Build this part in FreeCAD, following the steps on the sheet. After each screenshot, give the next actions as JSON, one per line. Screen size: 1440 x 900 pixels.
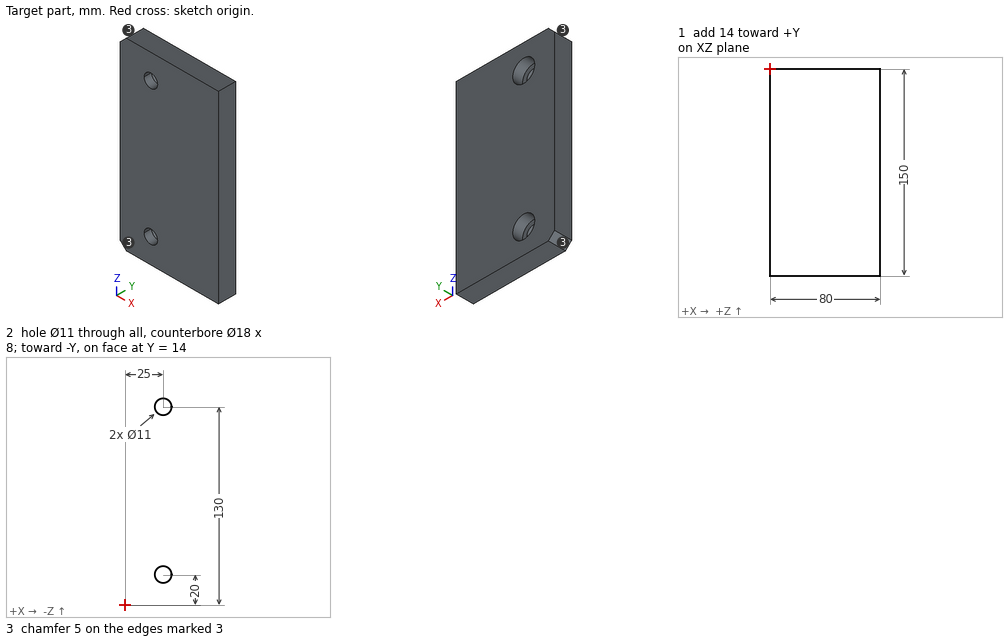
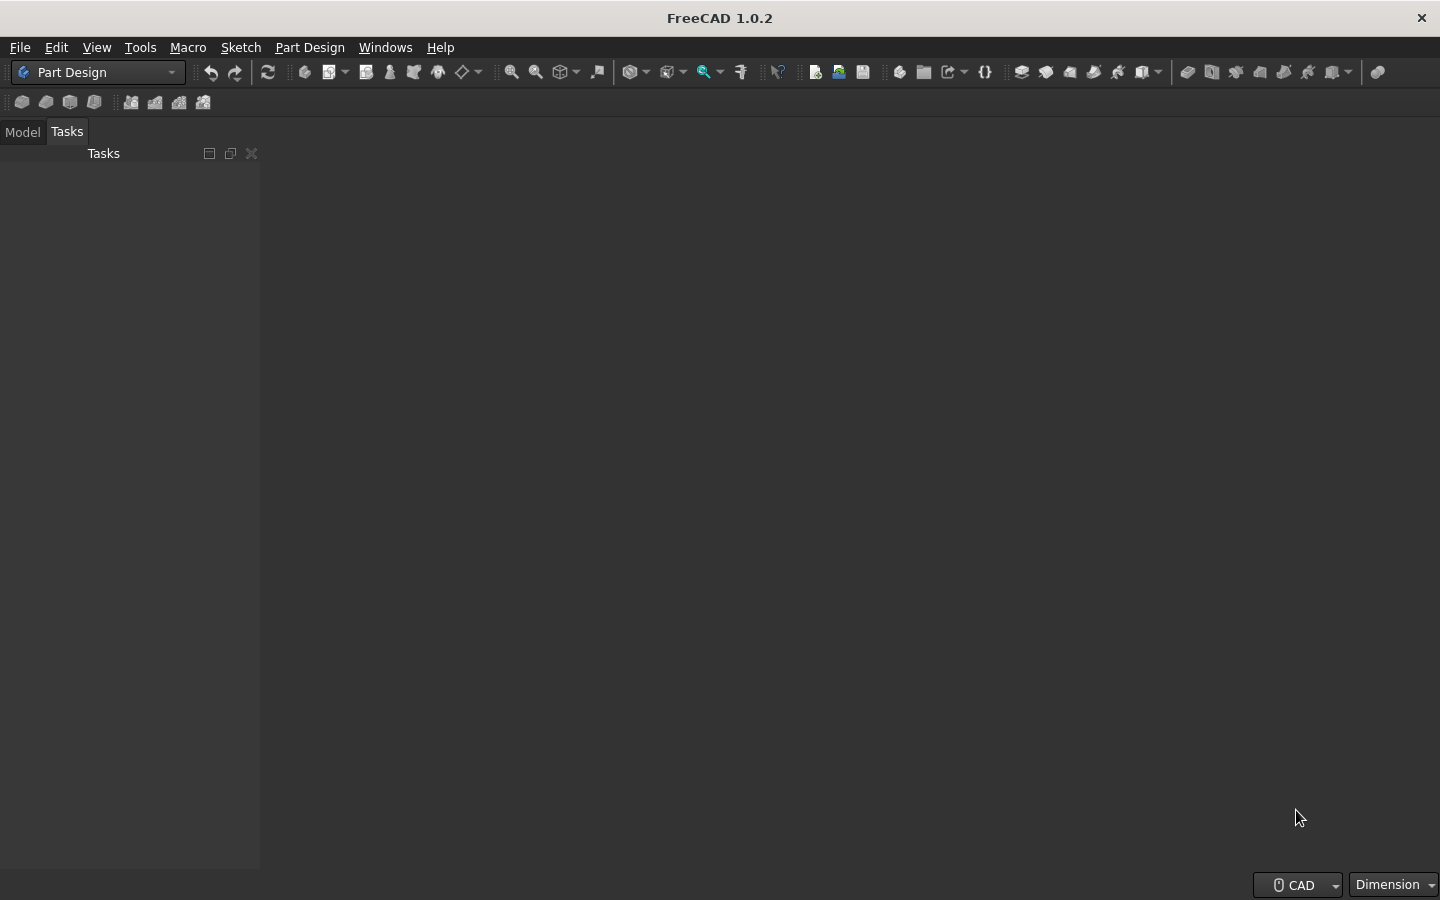
{"action": "key", "text": "ctrl+n"}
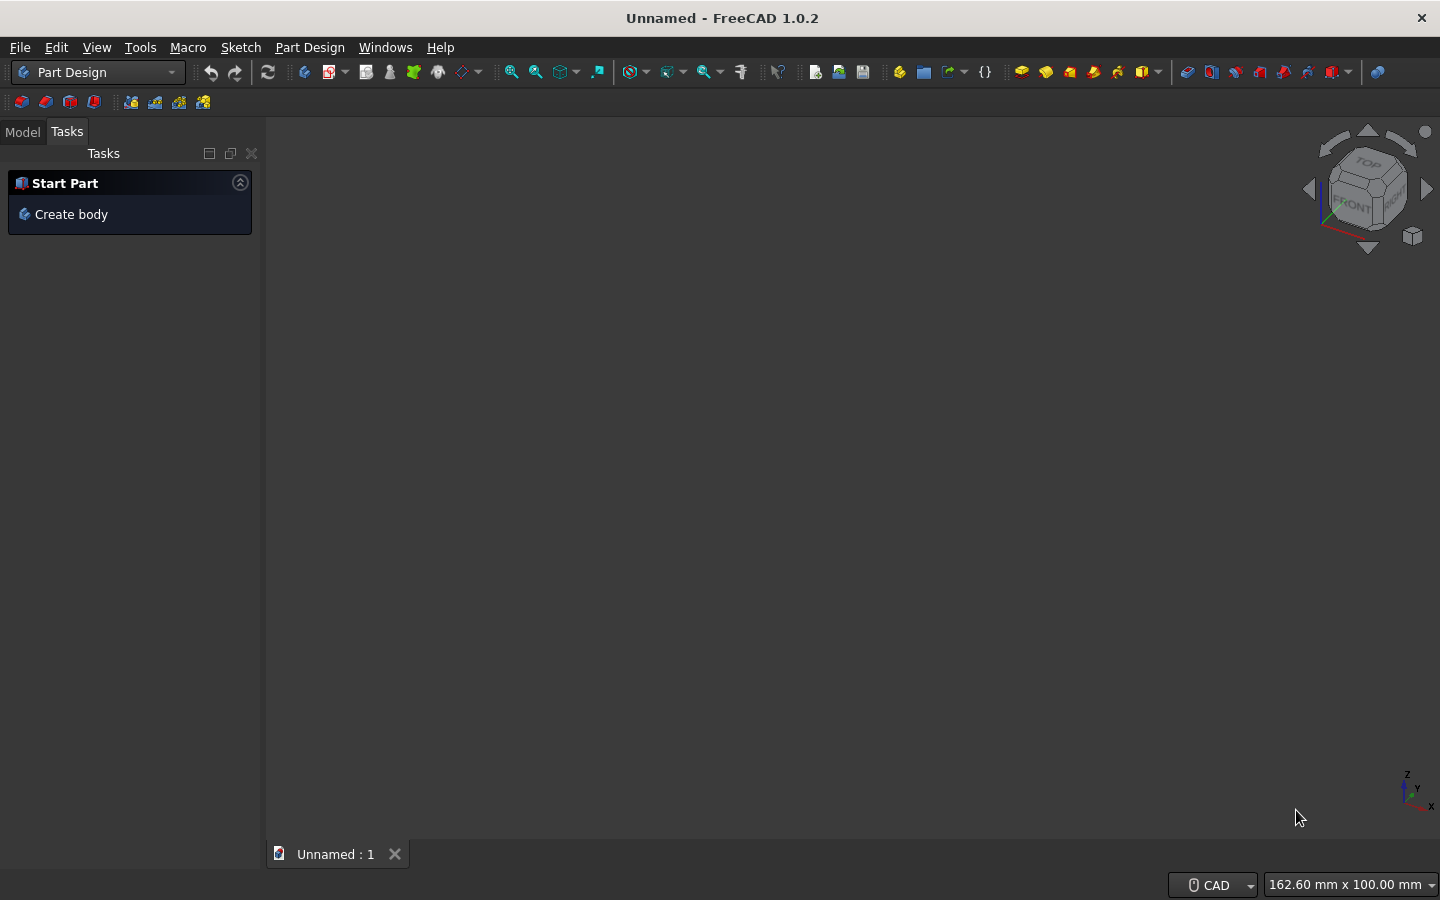
{"action": "left_click", "coordinate": [330, 72]}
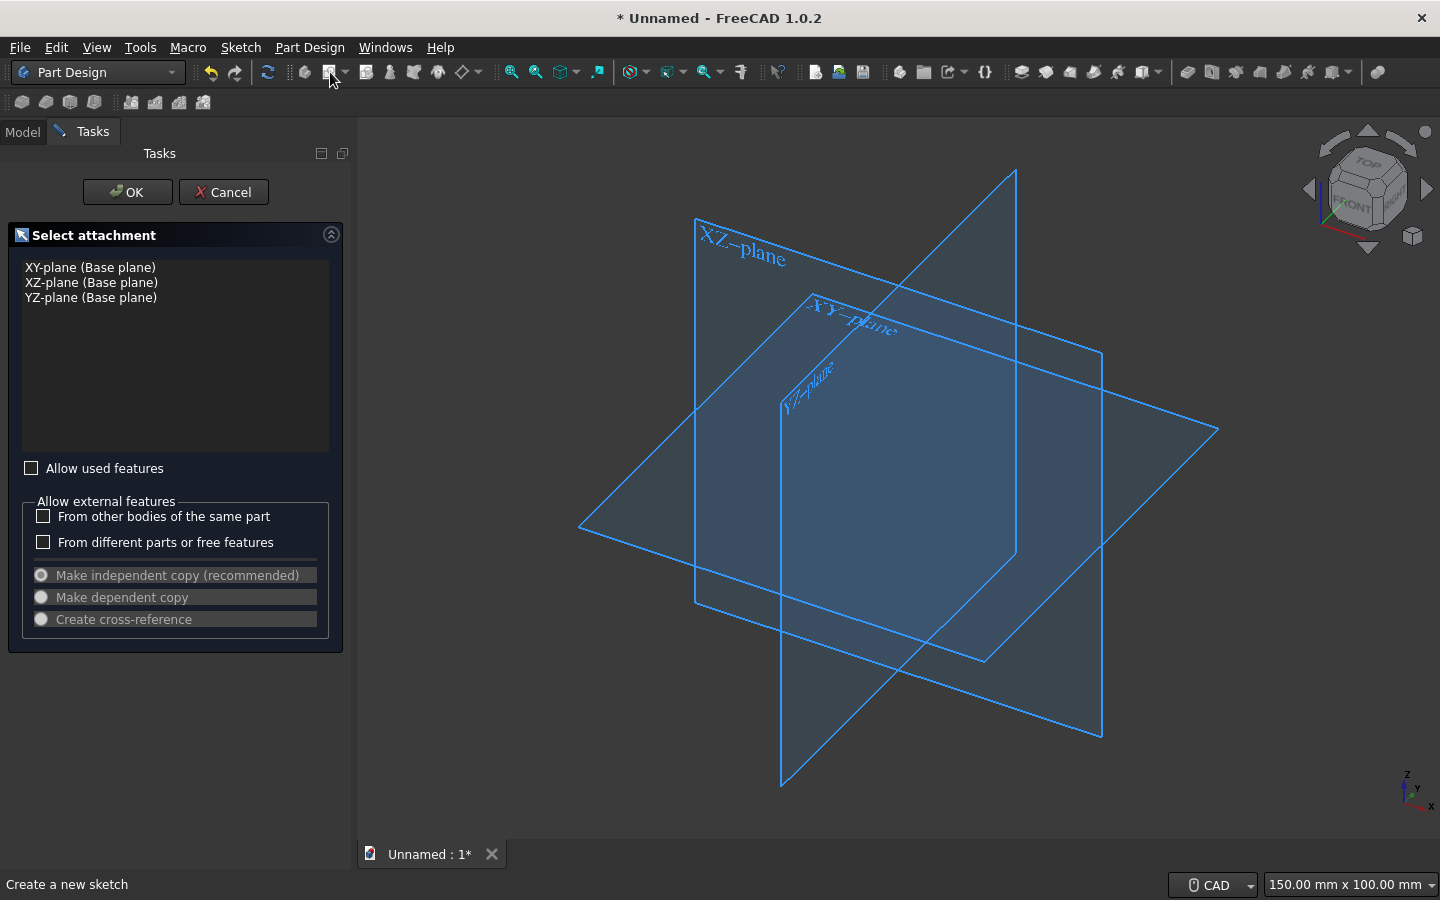
{"action": "left_click", "coordinate": [82, 282]}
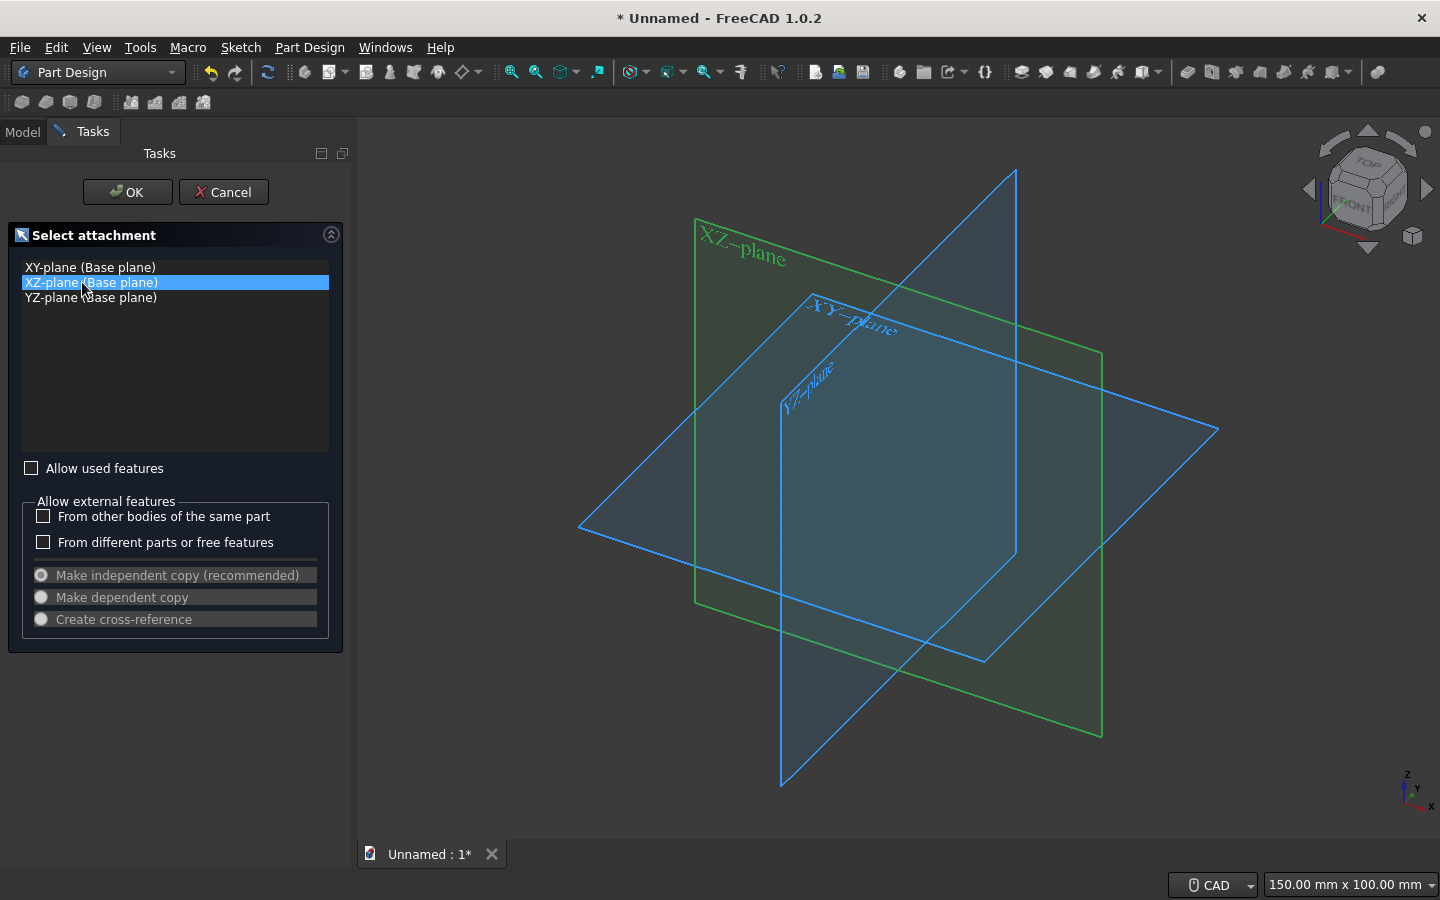
{"action": "left_click", "coordinate": [128, 192]}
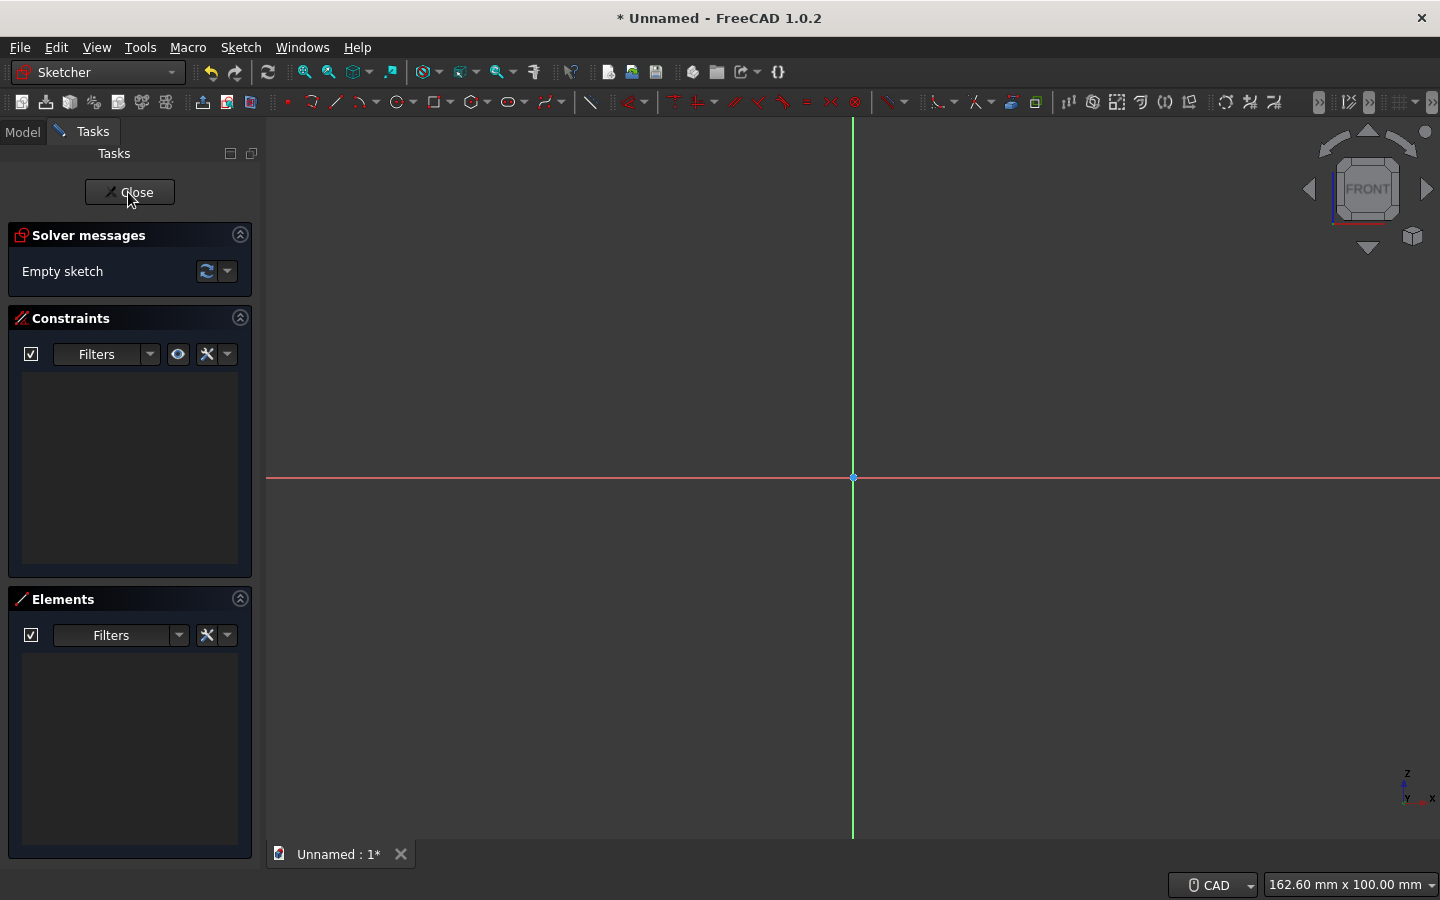
{"action": "scroll", "coordinate": [493, 145], "scroll_direction": "down", "scroll_amount": 4}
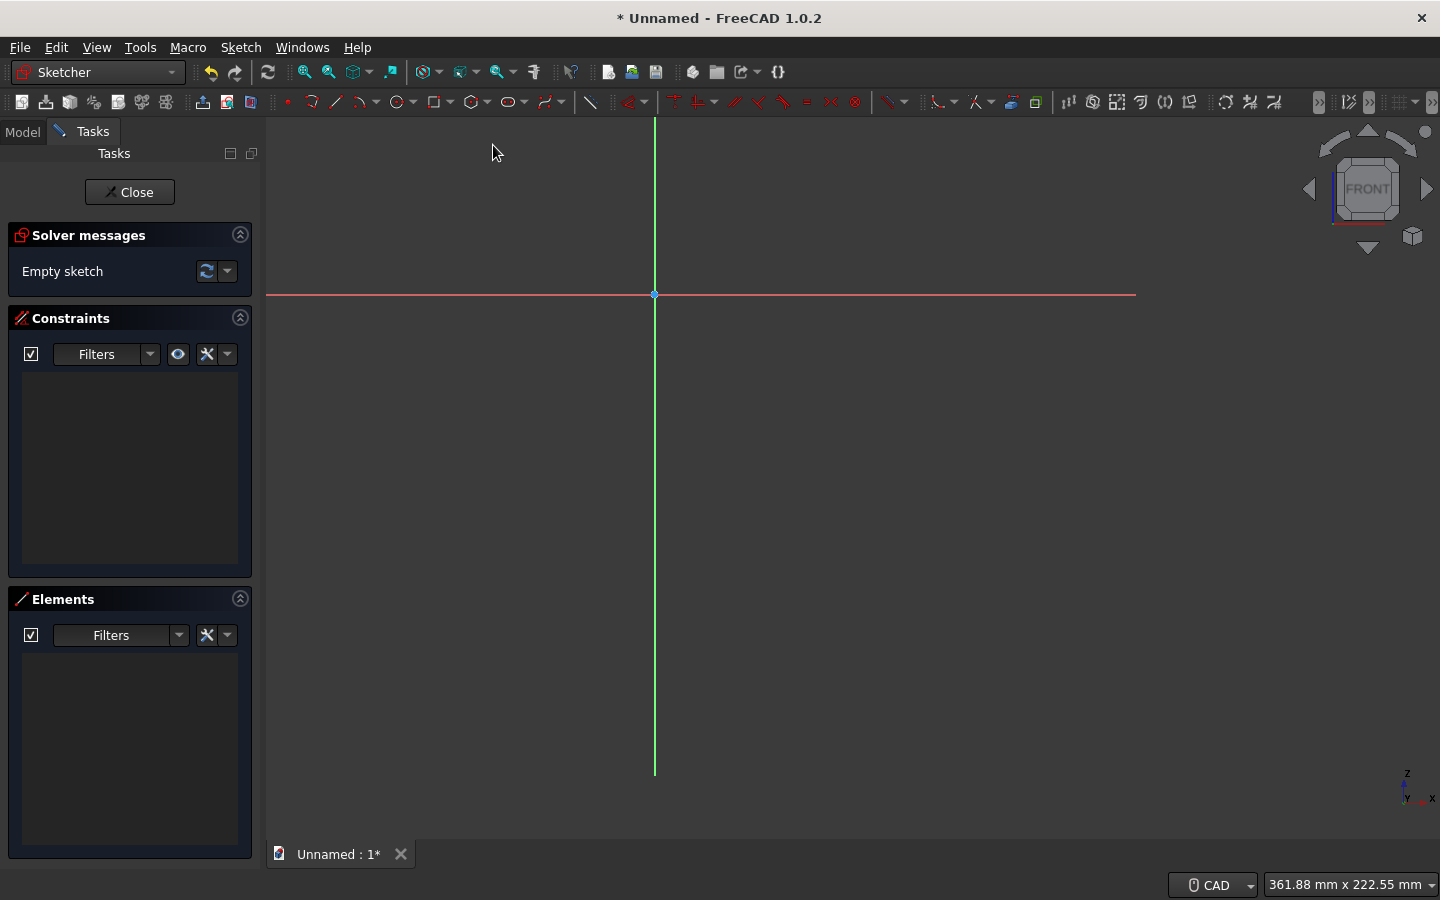
{"action": "left_click", "coordinate": [434, 102]}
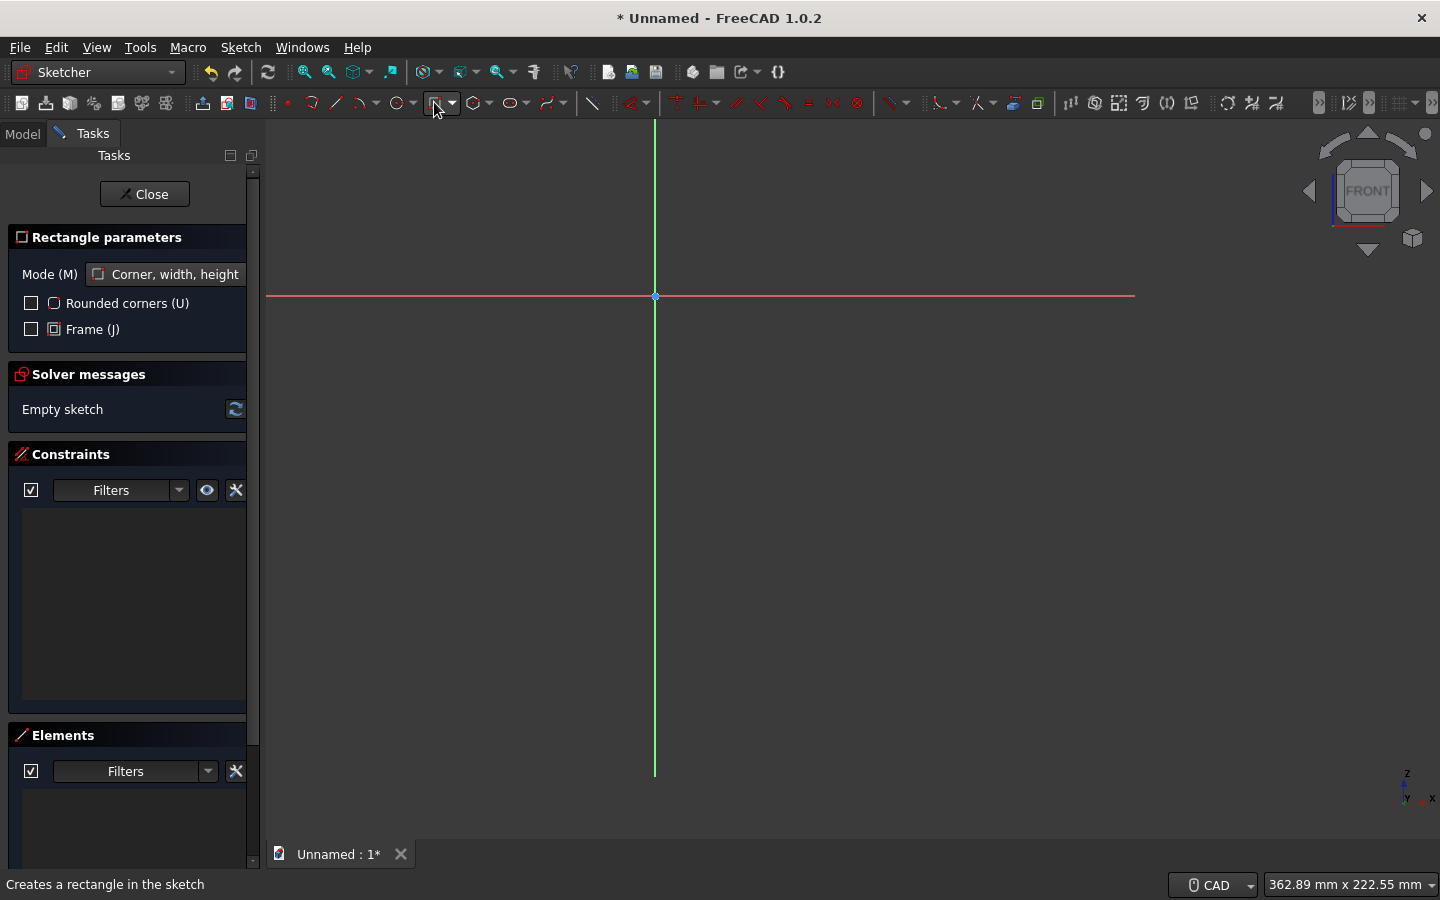
{"action": "left_click", "coordinate": [655, 296]}
{"action": "mouse_move", "coordinate": [914, 781]}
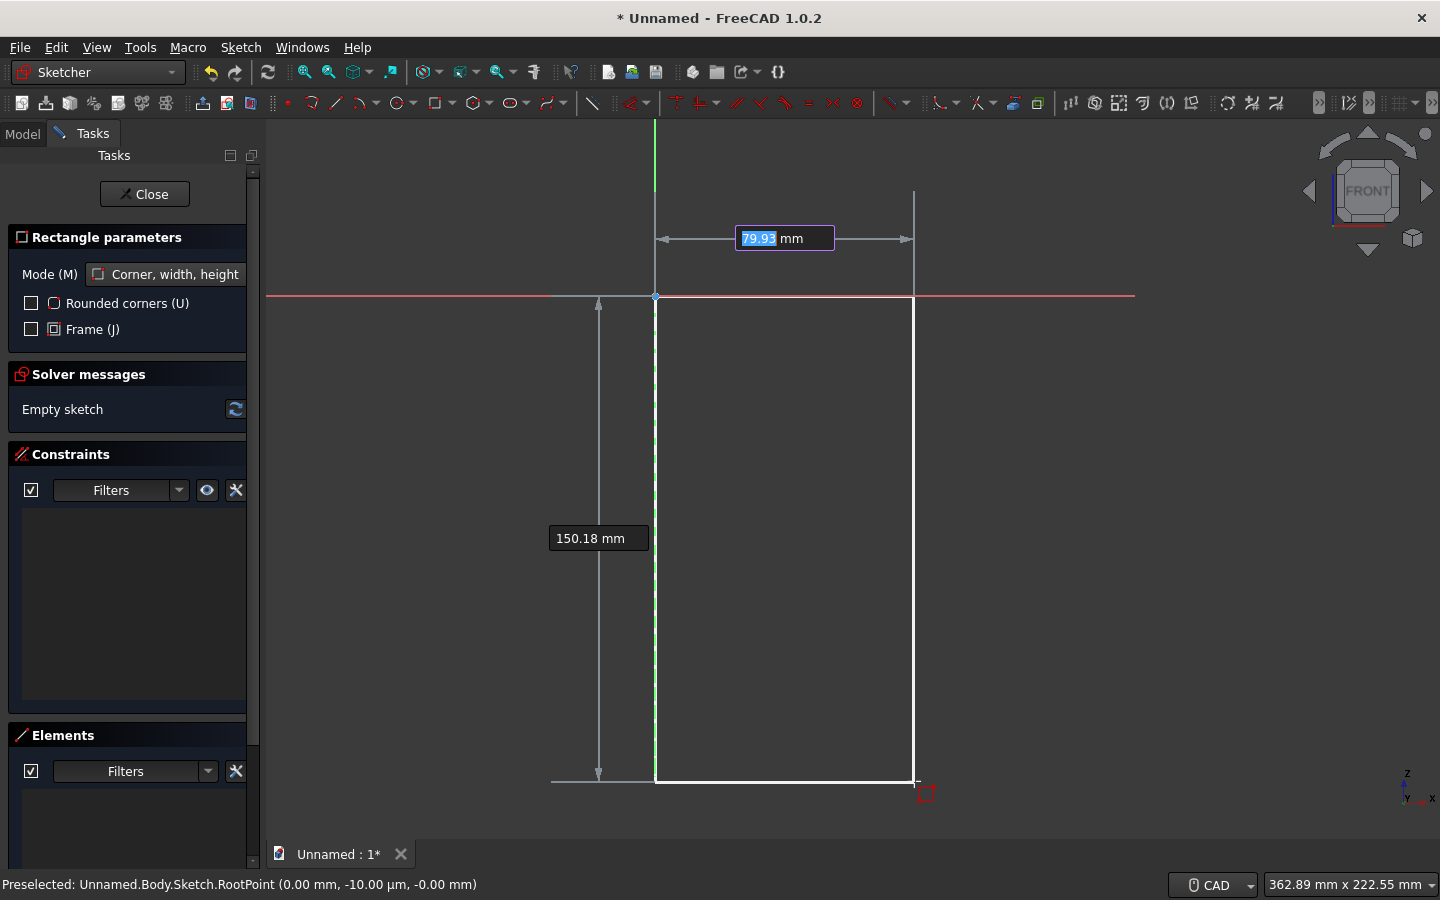
{"action": "type", "text": "80"}
{"action": "key", "text": "Tab"}
{"action": "type", "text": "150"}
{"action": "key", "text": "Return"}
{"action": "key", "text": "Escape"}